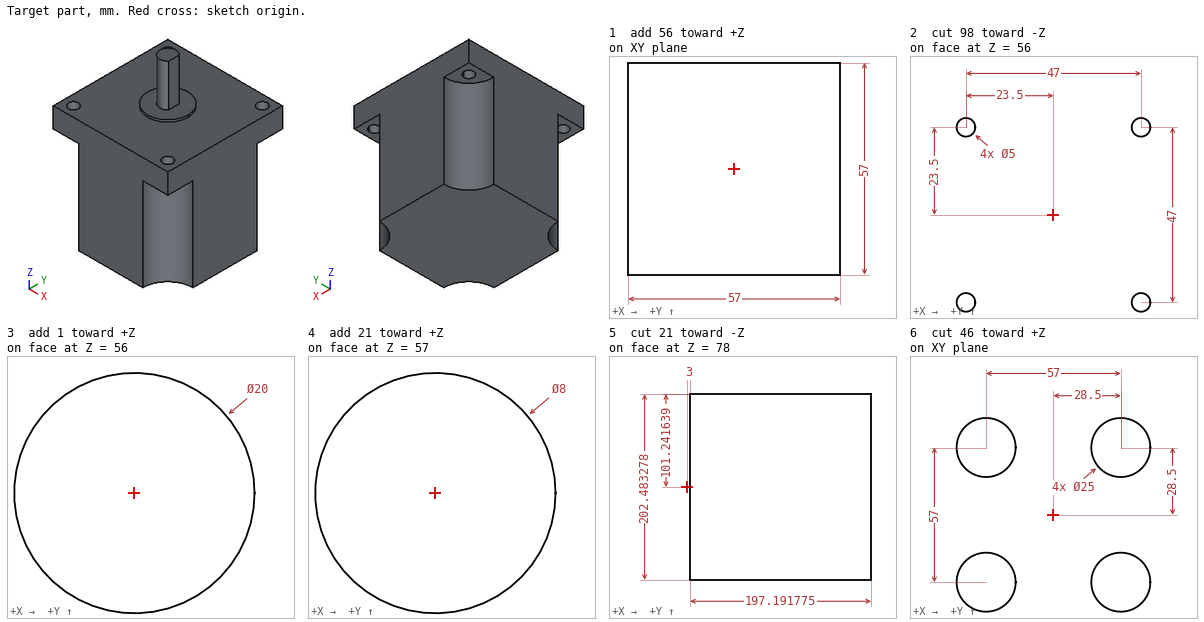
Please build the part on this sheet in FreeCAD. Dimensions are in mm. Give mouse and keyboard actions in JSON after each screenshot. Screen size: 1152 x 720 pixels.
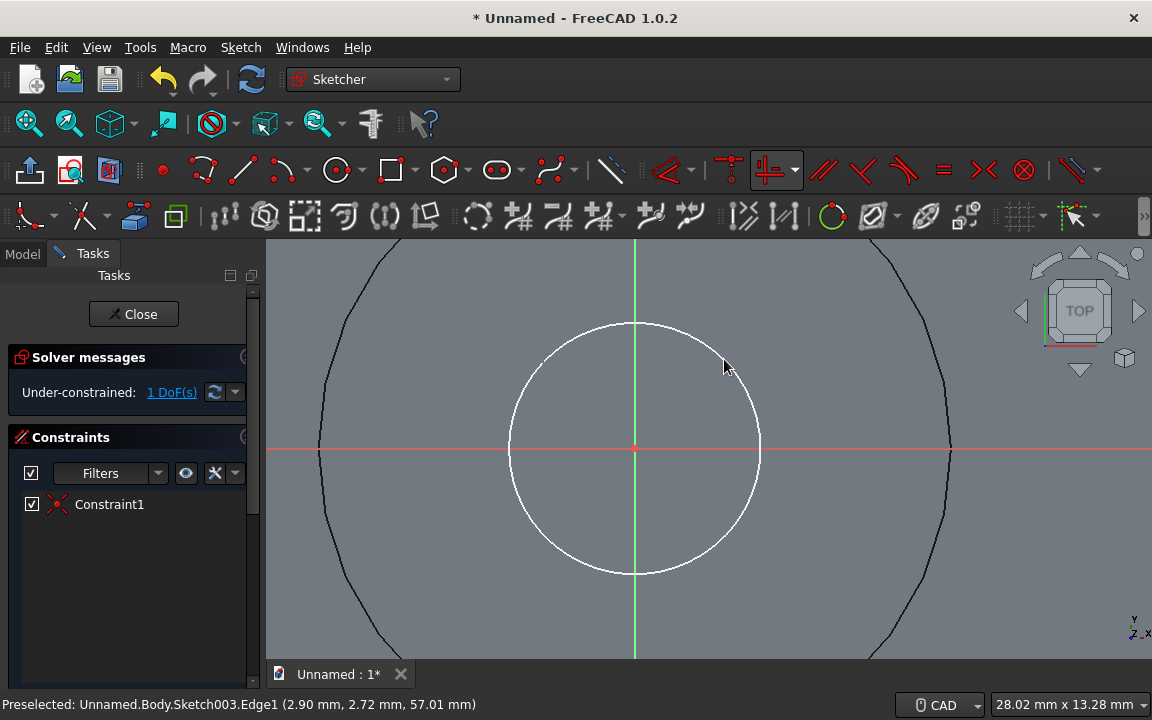
{"action": "left_click", "coordinate": [666, 170]}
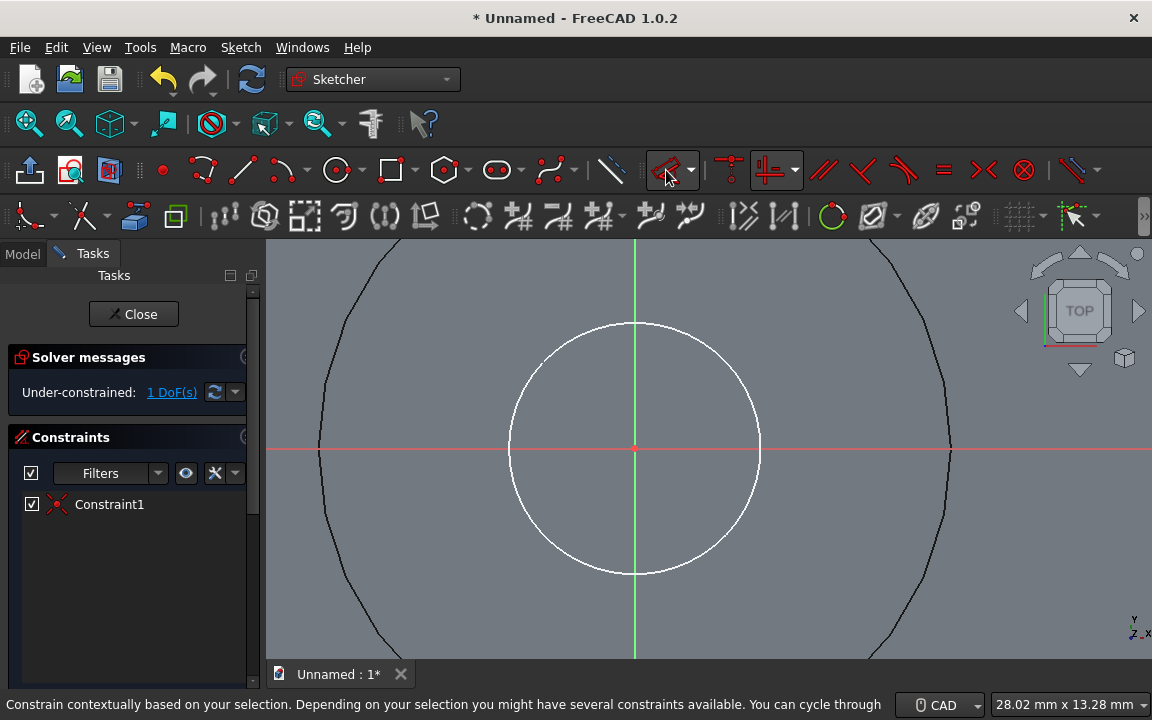
{"action": "left_click", "coordinate": [723, 359]}
{"action": "left_click", "coordinate": [745, 336]}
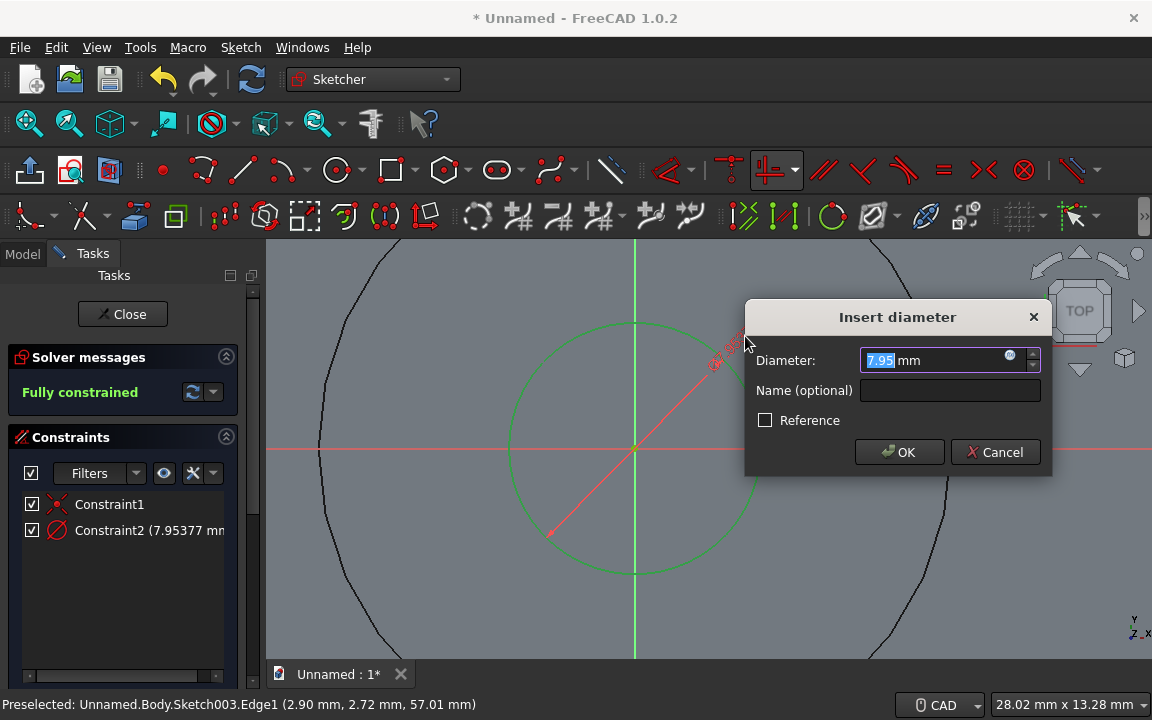
{"action": "type", "text": "8"}
{"action": "key", "text": "Return"}
{"action": "key", "text": "Escape"}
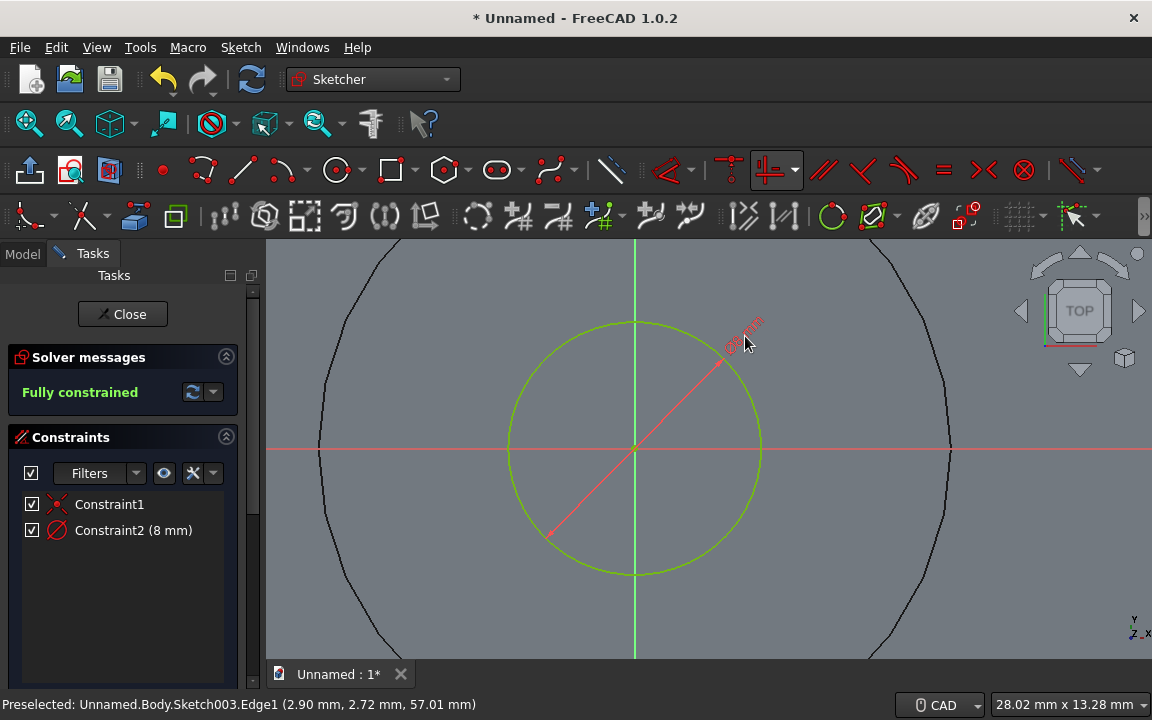
{"action": "left_click", "coordinate": [123, 314]}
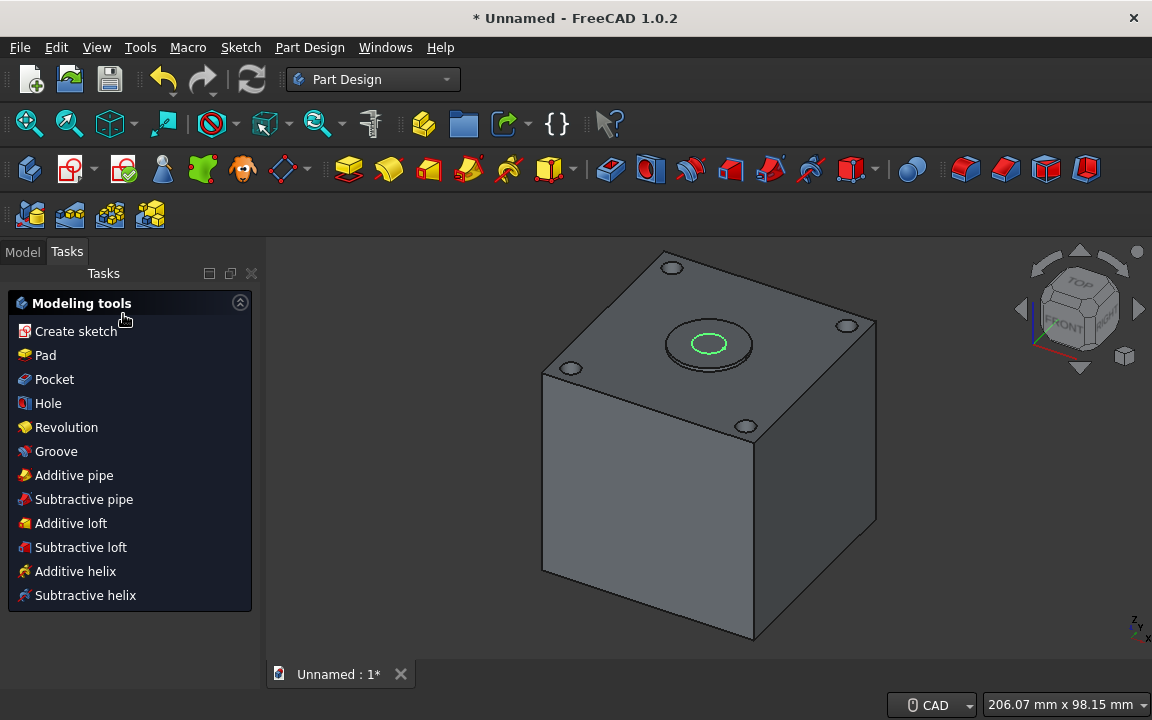
{"action": "left_click", "coordinate": [350, 170]}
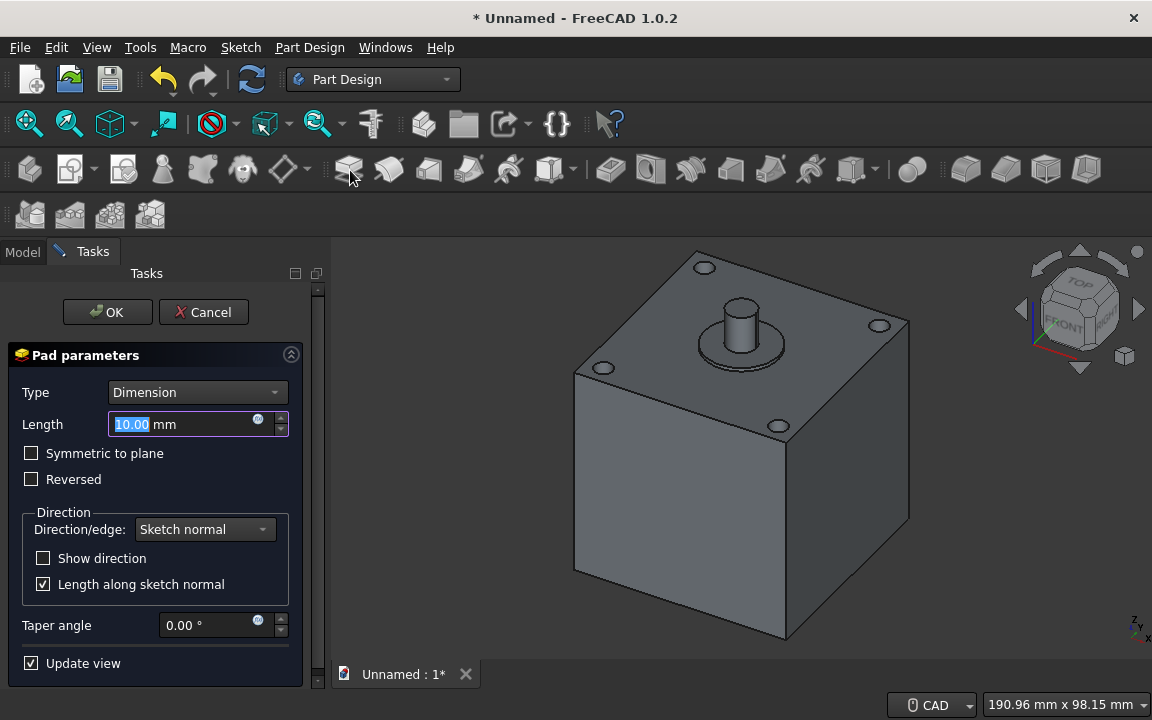
{"action": "type", "text": "21"}
{"action": "key", "text": "Tab"}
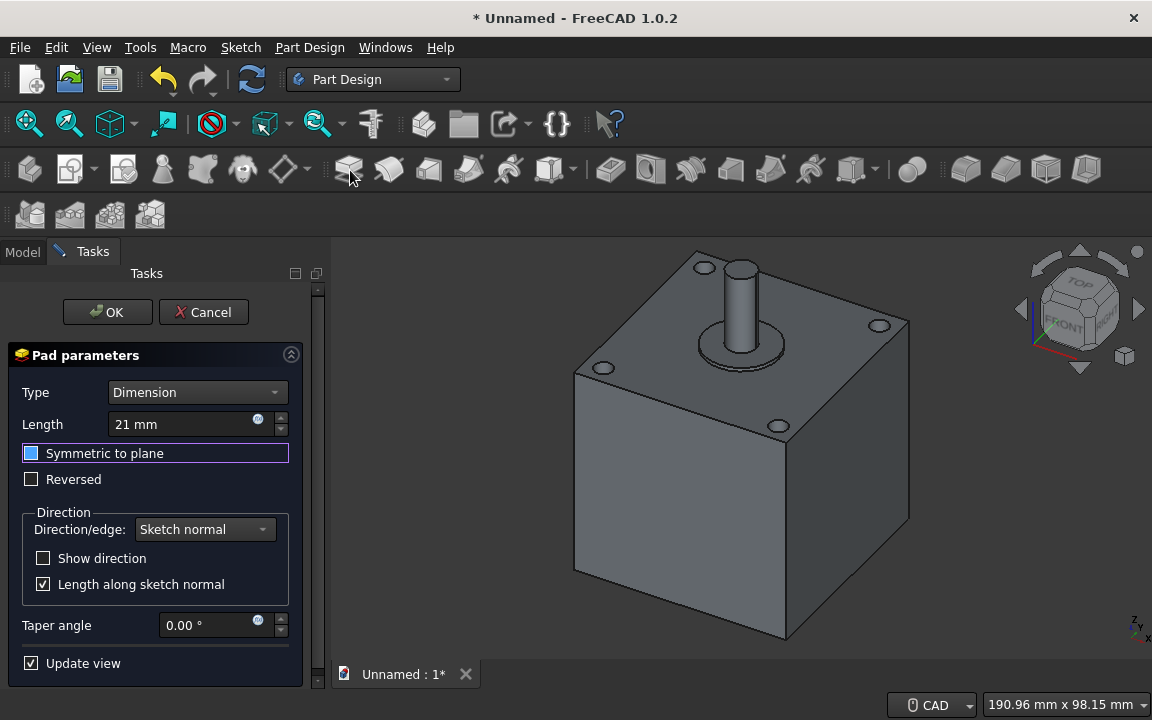
{"action": "left_click", "coordinate": [108, 312]}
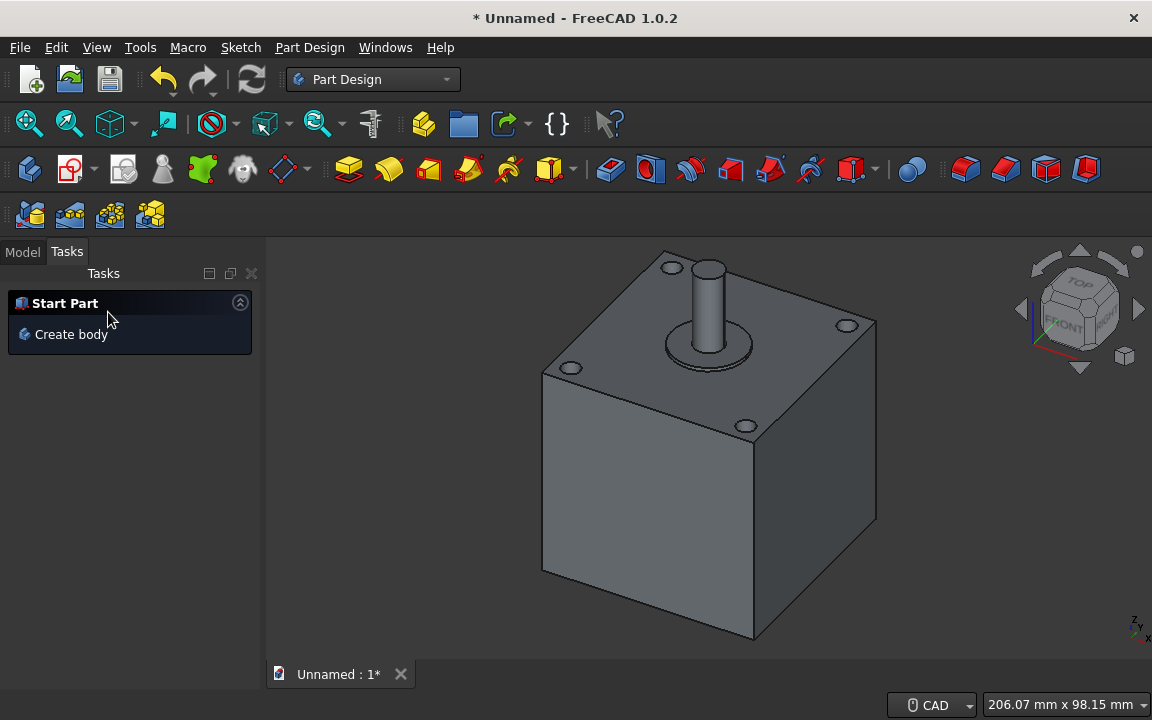
{"action": "left_click", "coordinate": [30, 124]}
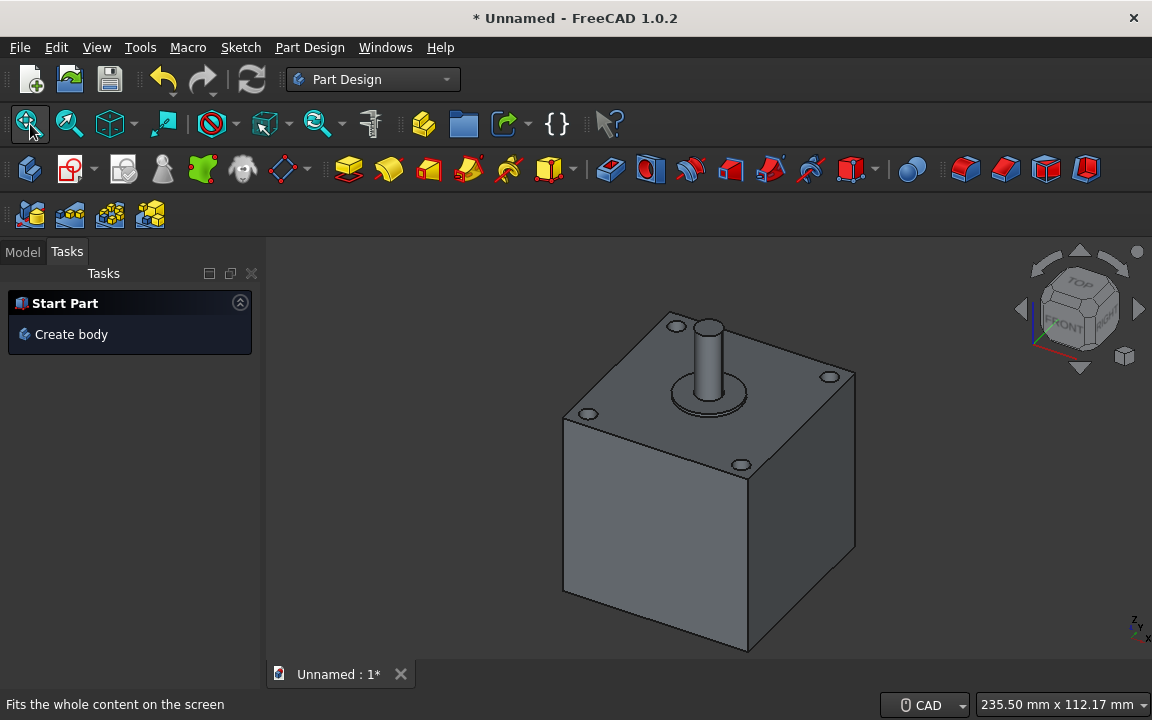
{"action": "left_click", "coordinate": [709, 327]}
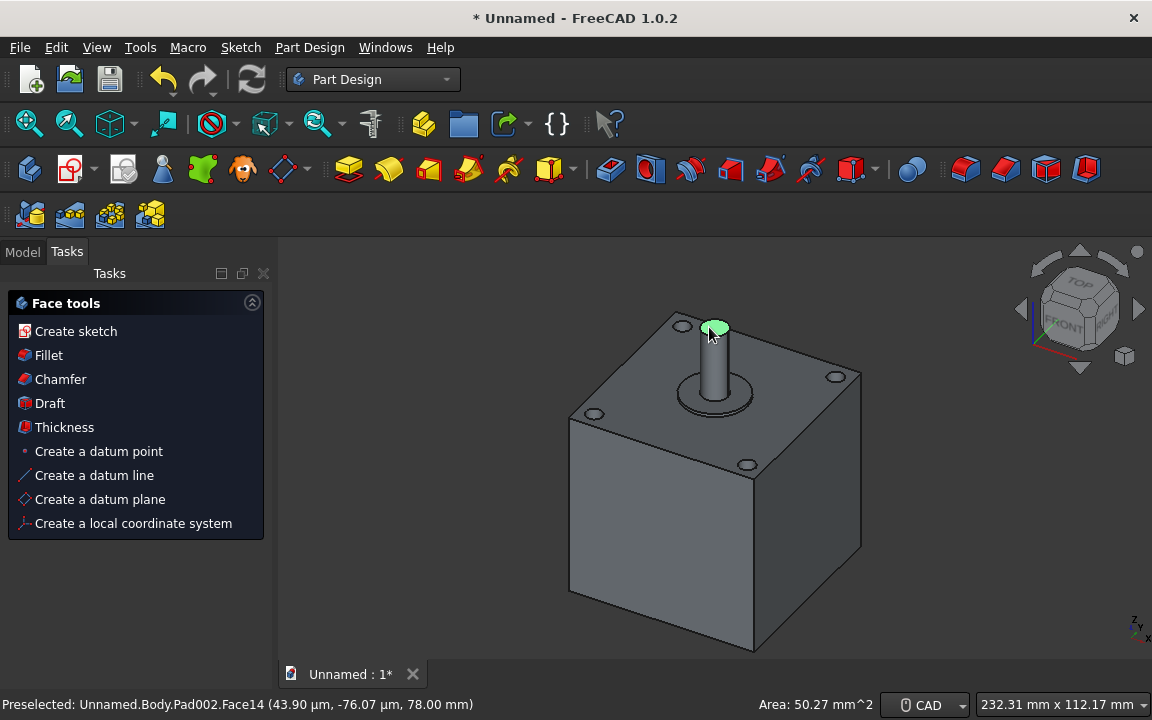
{"action": "left_click", "coordinate": [70, 170]}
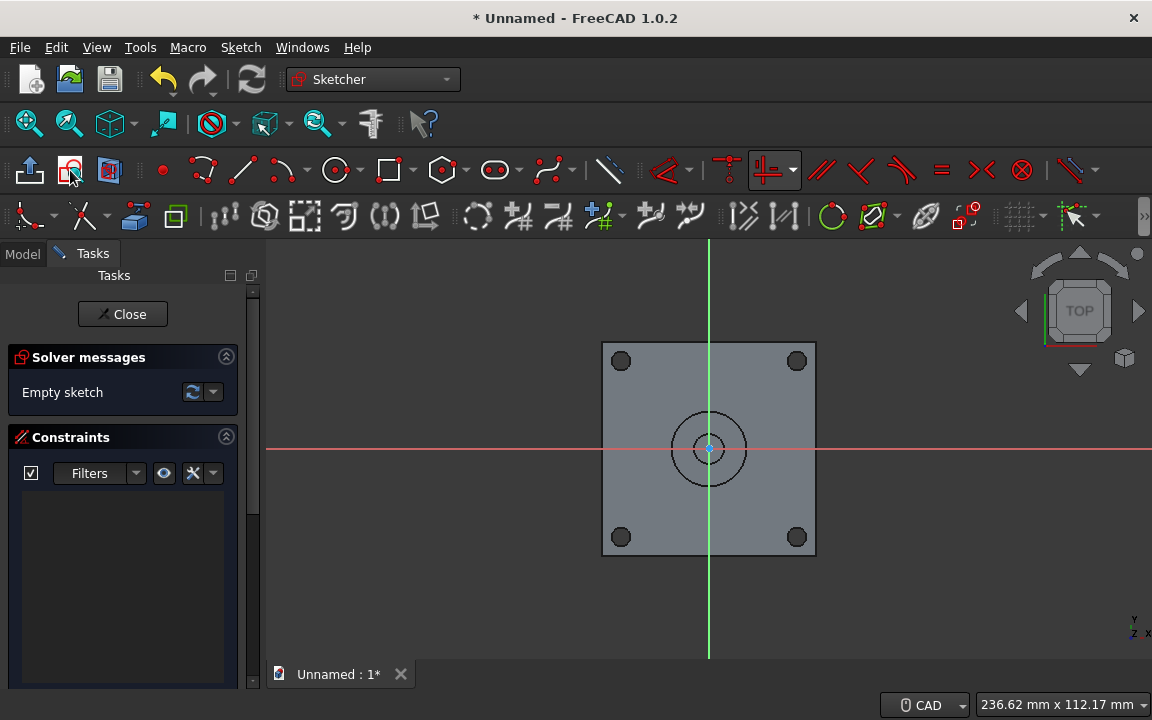
{"action": "scroll", "coordinate": [383, 449], "scroll_direction": "down", "scroll_amount": 5}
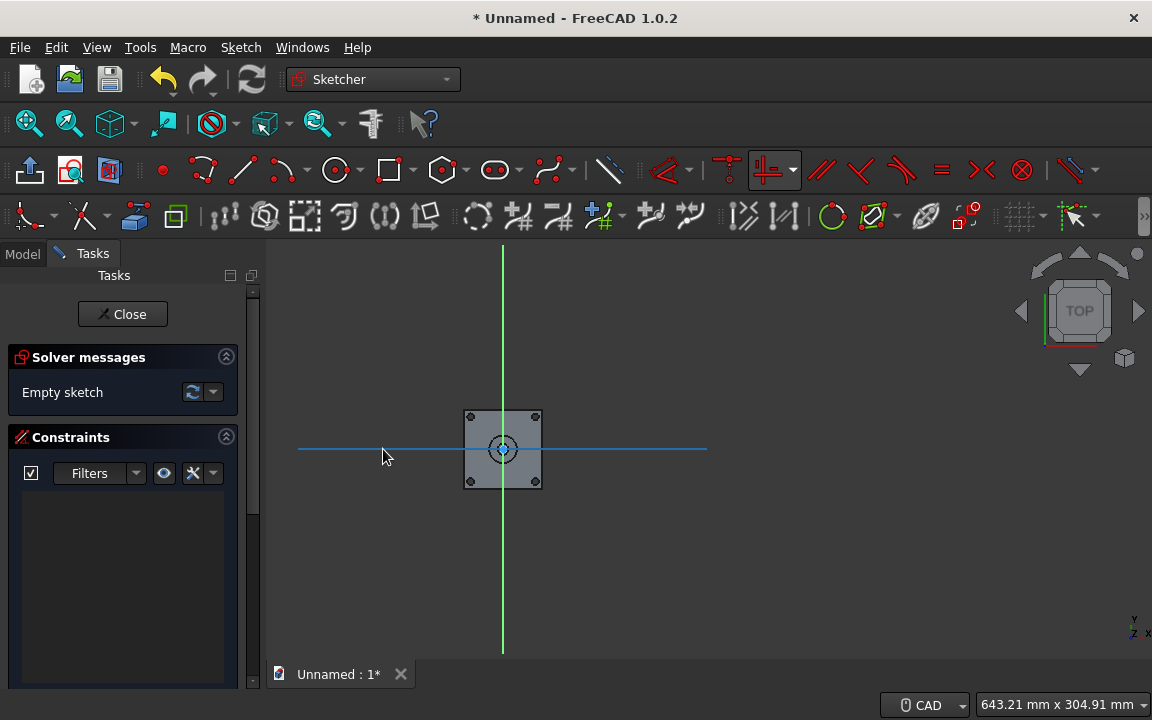
{"action": "left_click", "coordinate": [390, 170]}